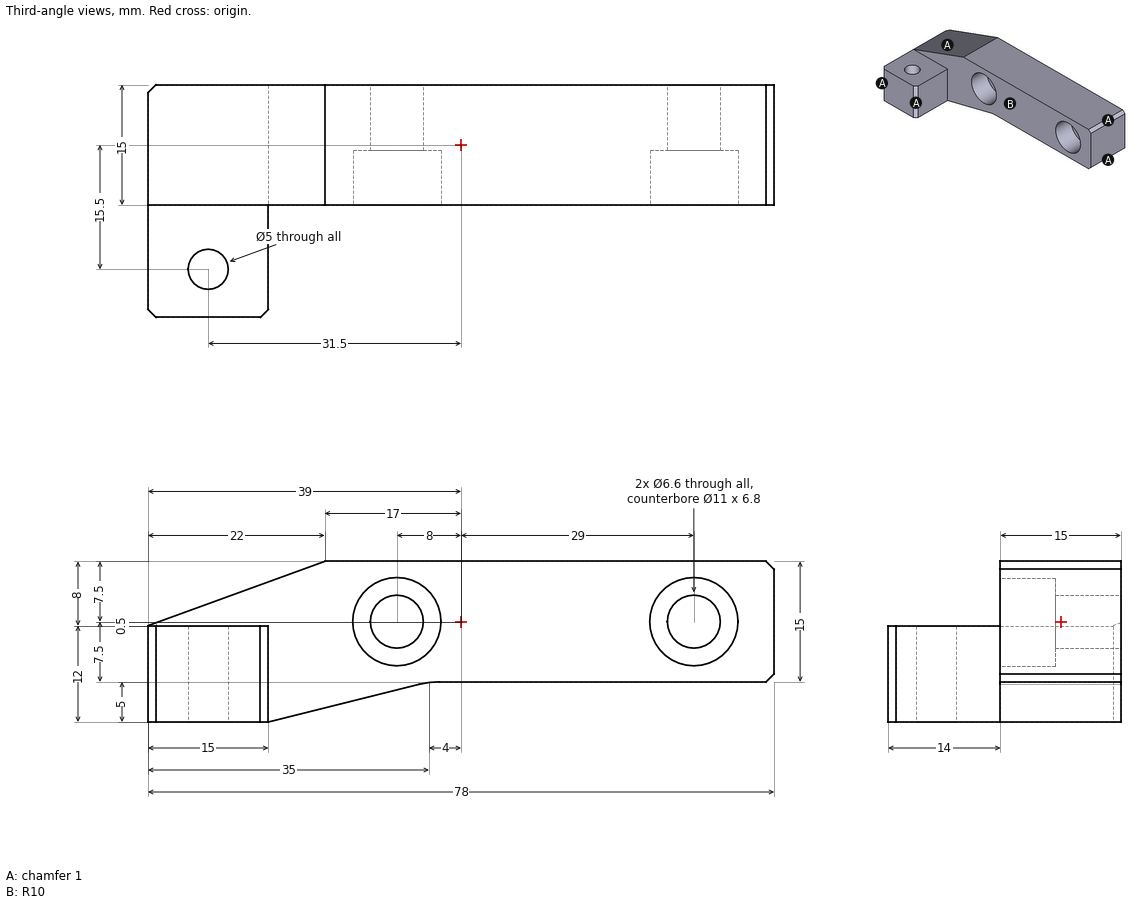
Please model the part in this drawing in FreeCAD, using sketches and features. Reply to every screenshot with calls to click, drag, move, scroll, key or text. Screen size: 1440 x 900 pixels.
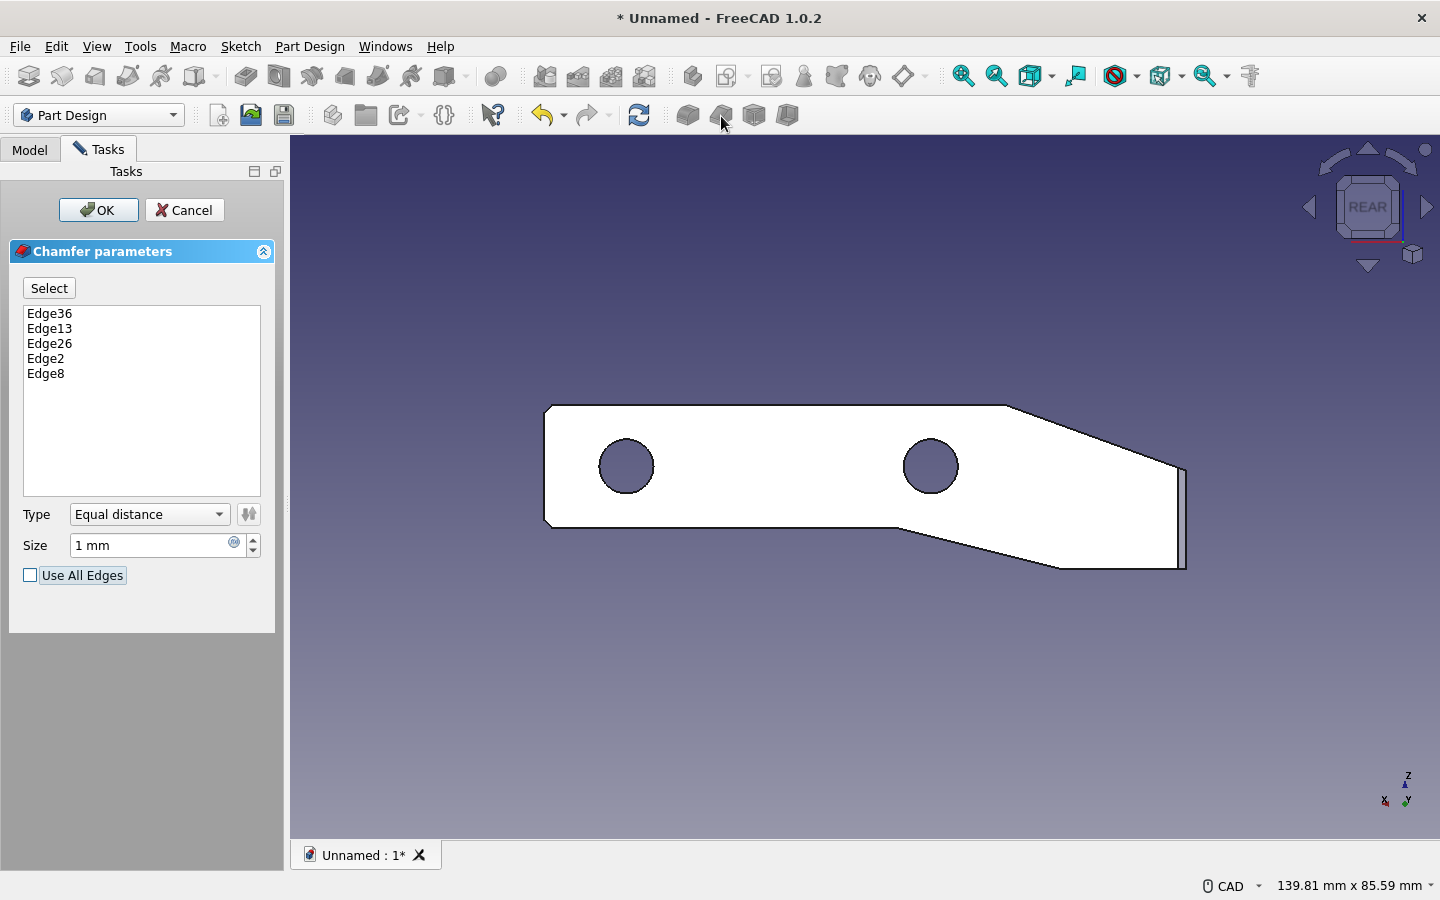
click(99, 210)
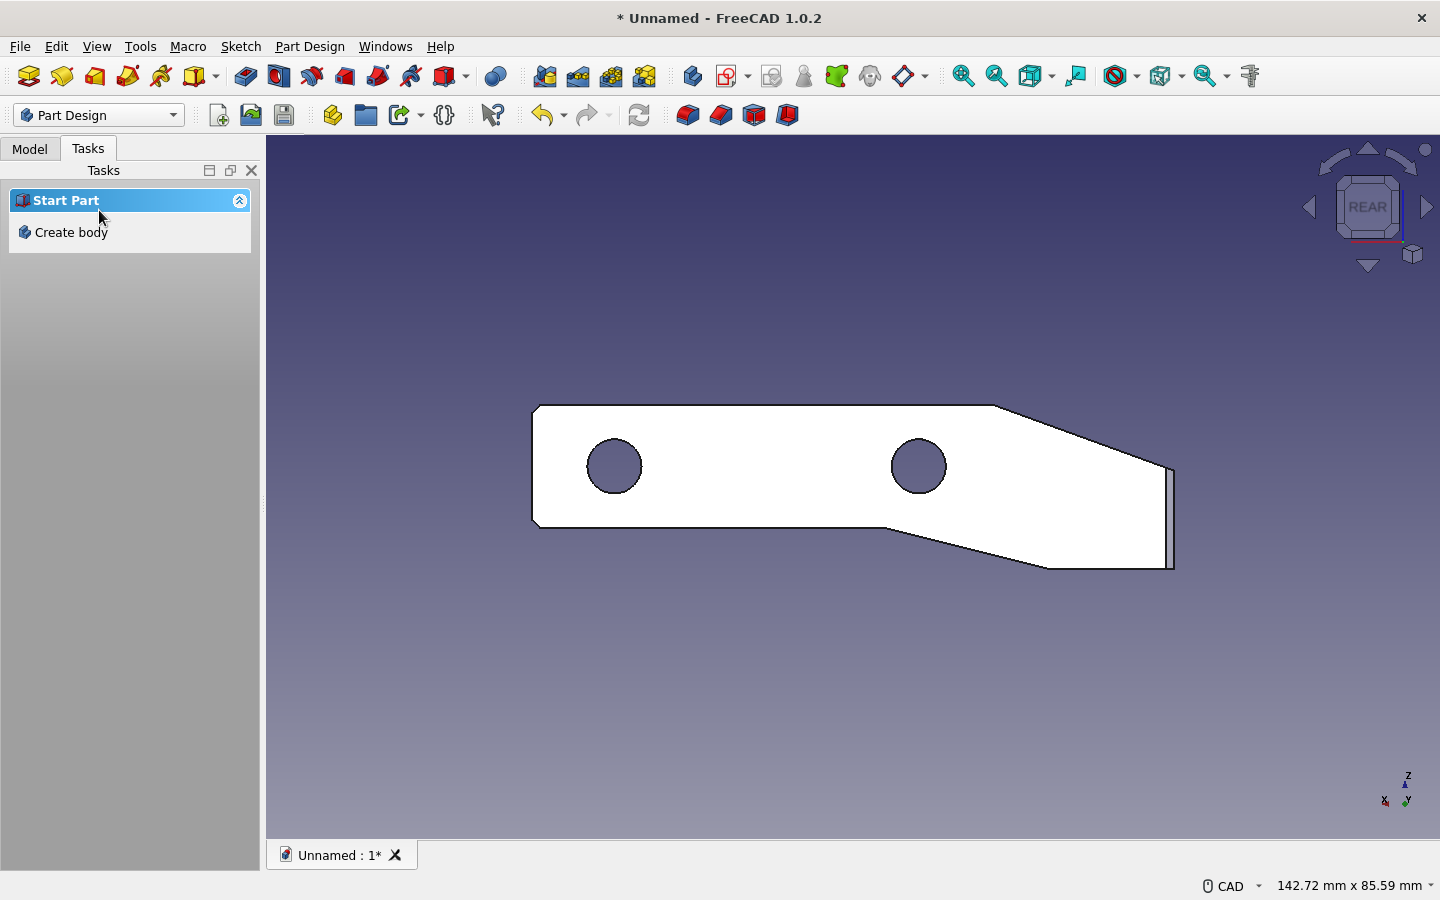
key(0)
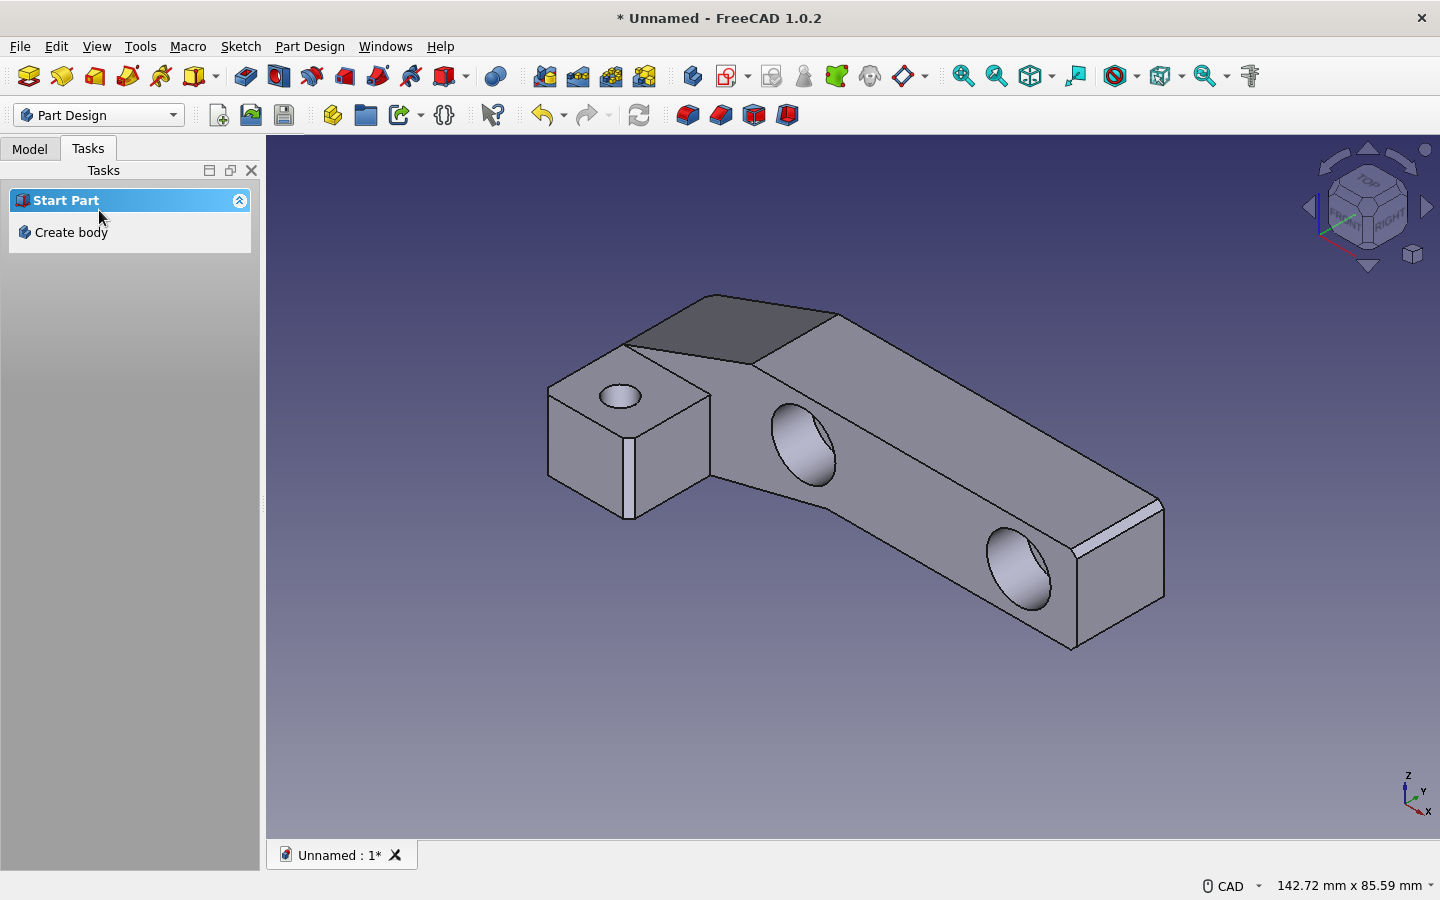
key(2)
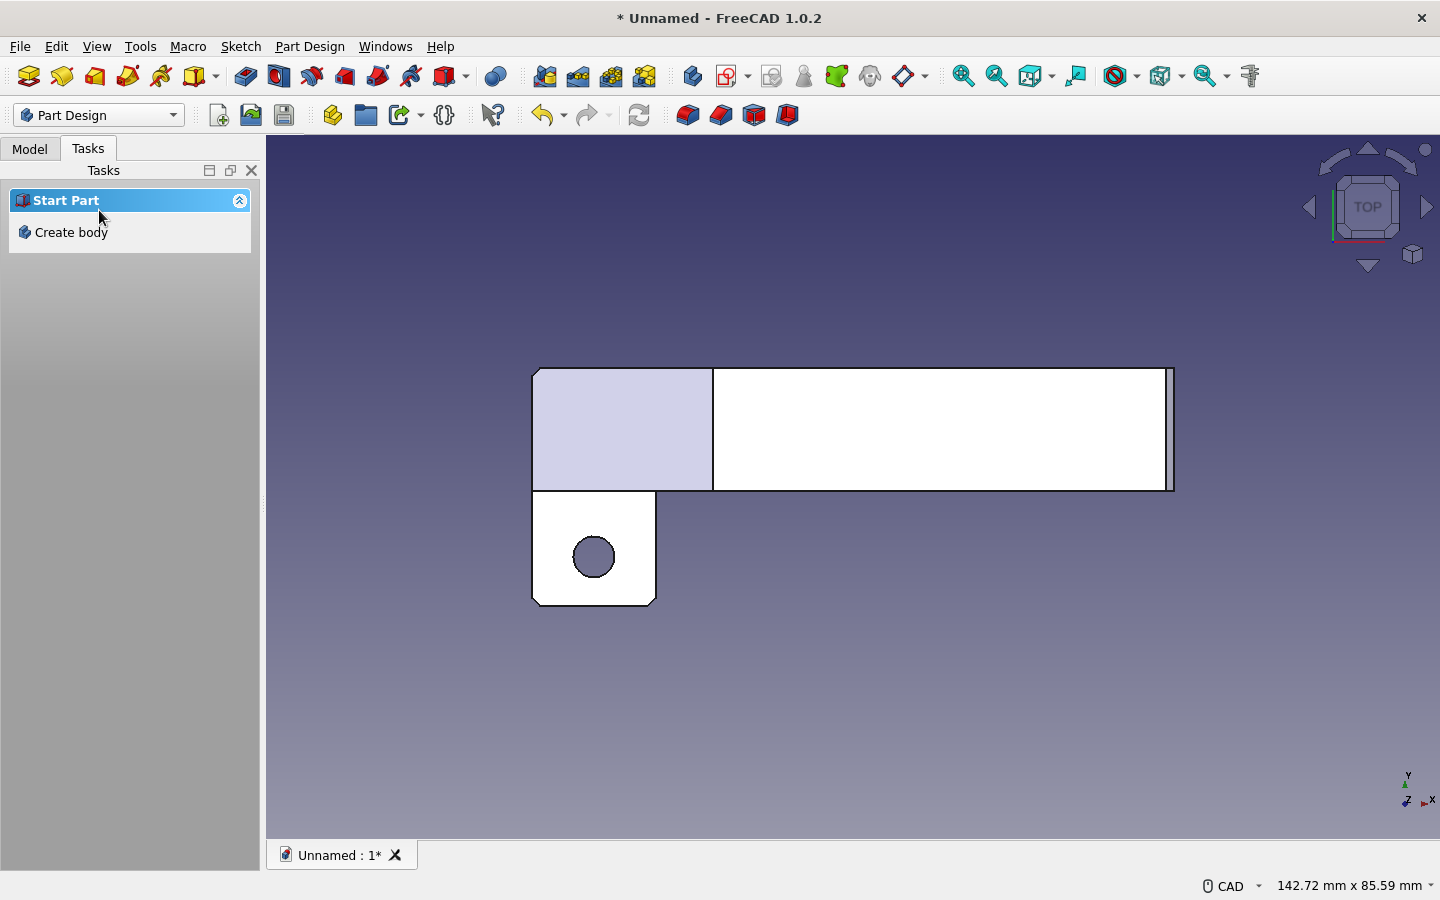
key(1)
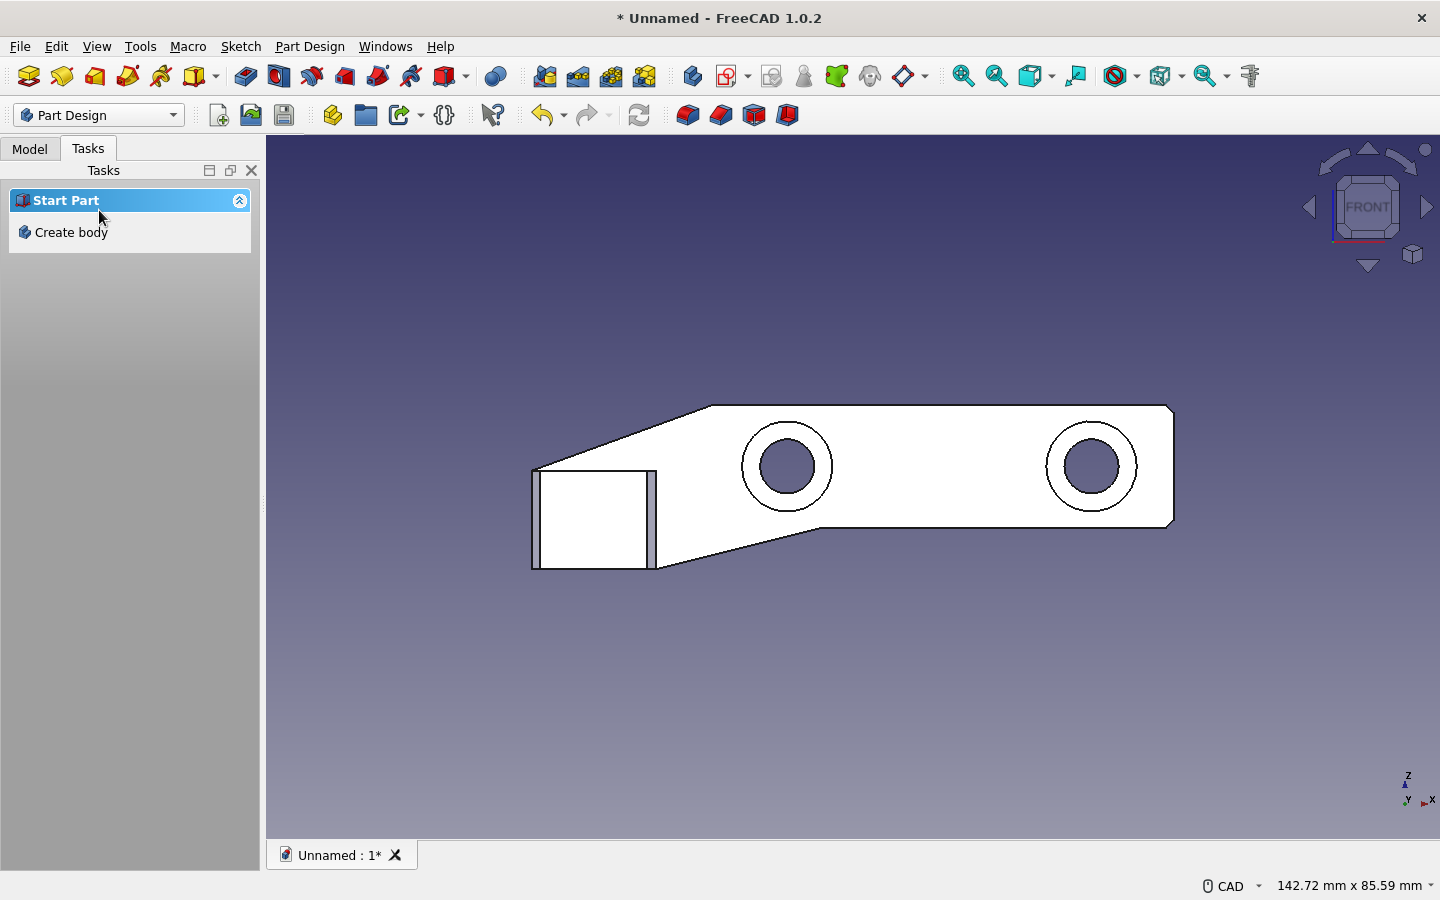
key(3)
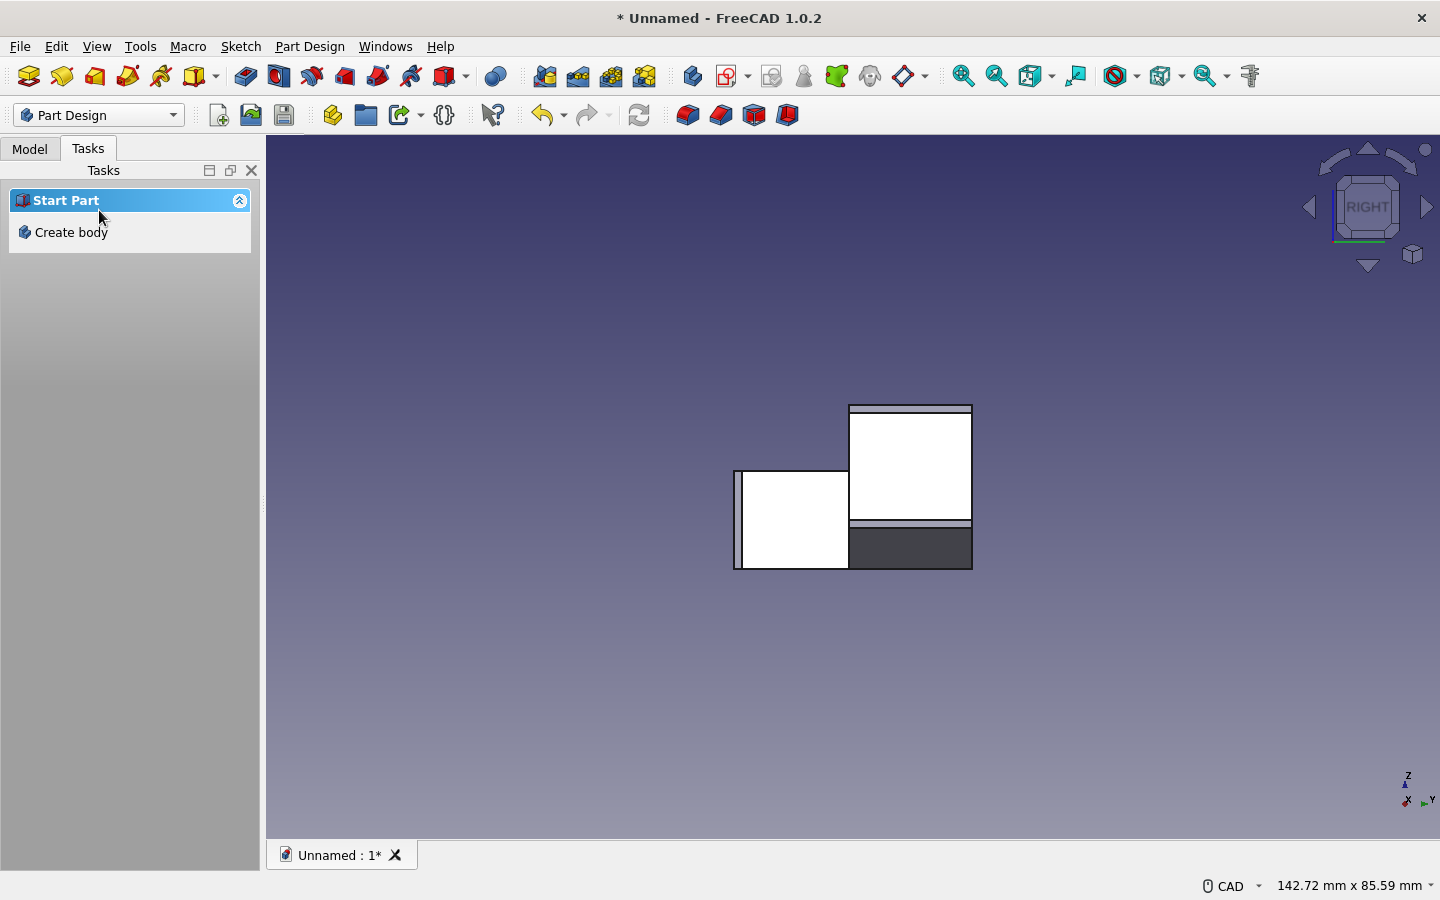
key(v)
key(f)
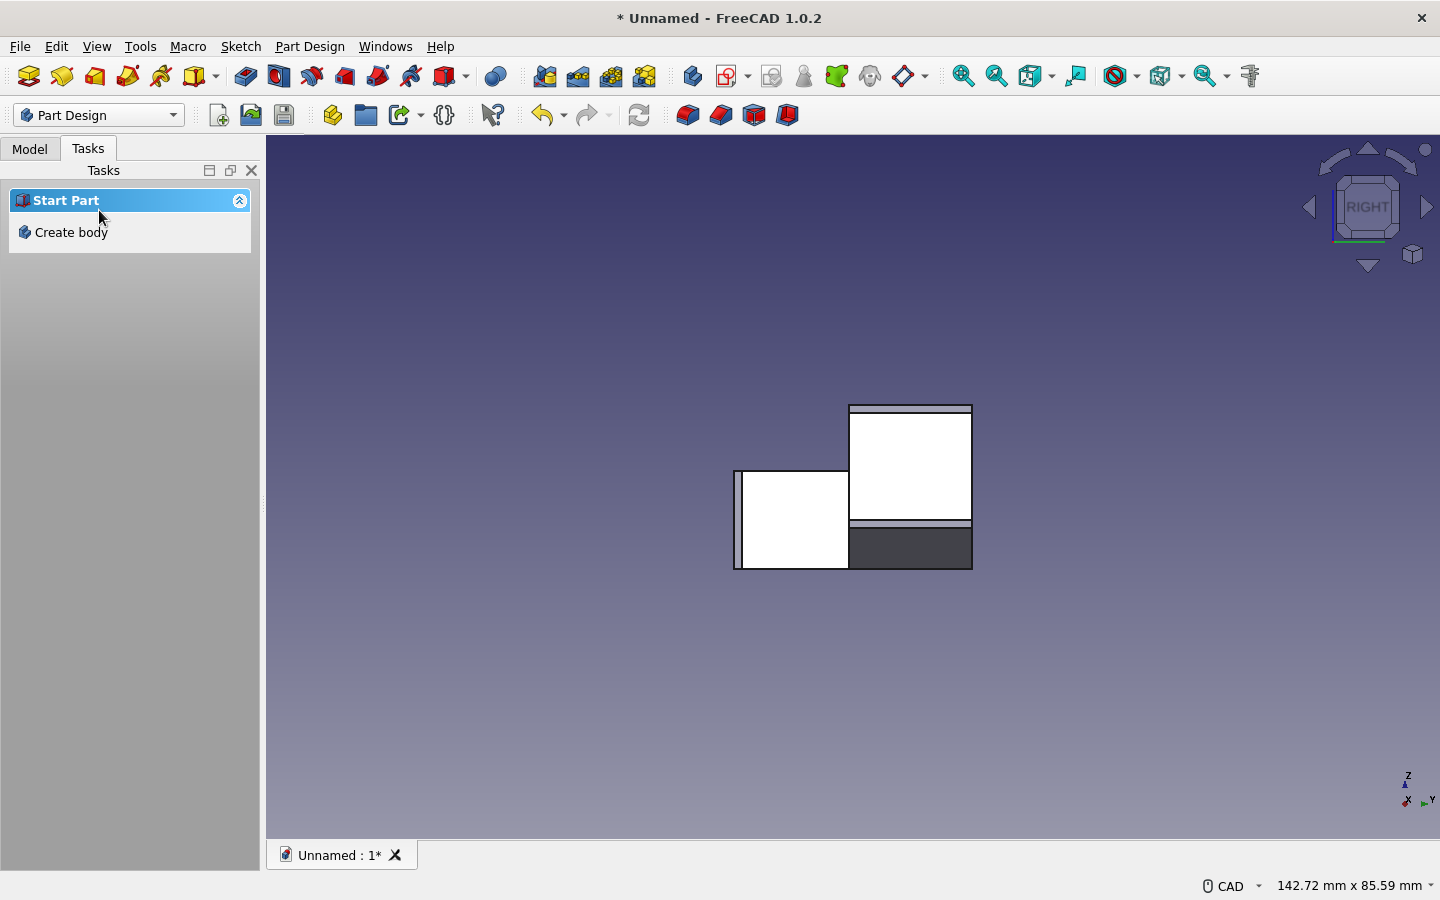
key(5)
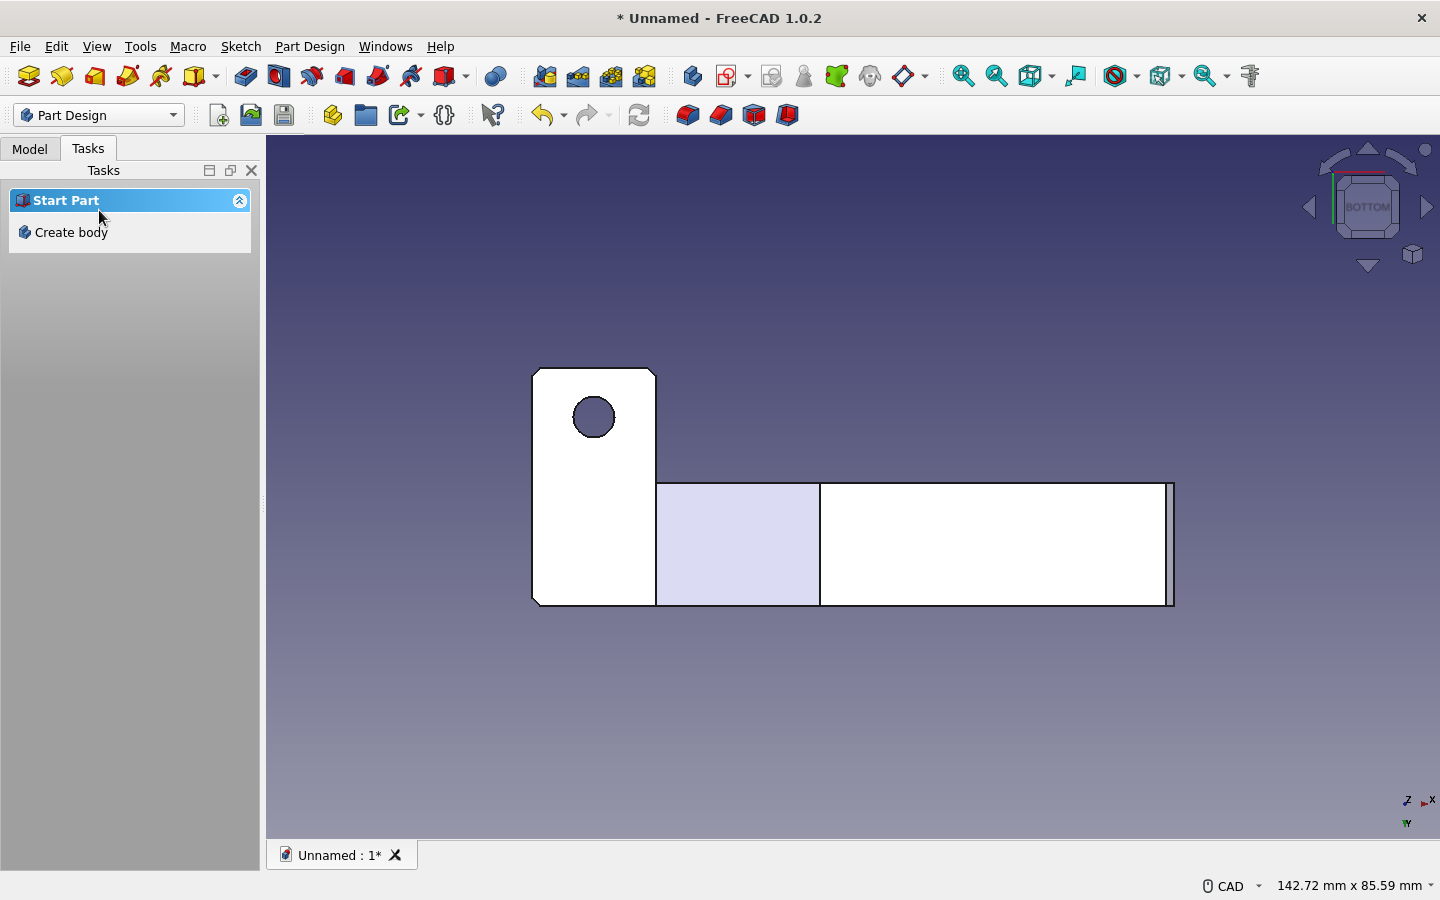
key(4)